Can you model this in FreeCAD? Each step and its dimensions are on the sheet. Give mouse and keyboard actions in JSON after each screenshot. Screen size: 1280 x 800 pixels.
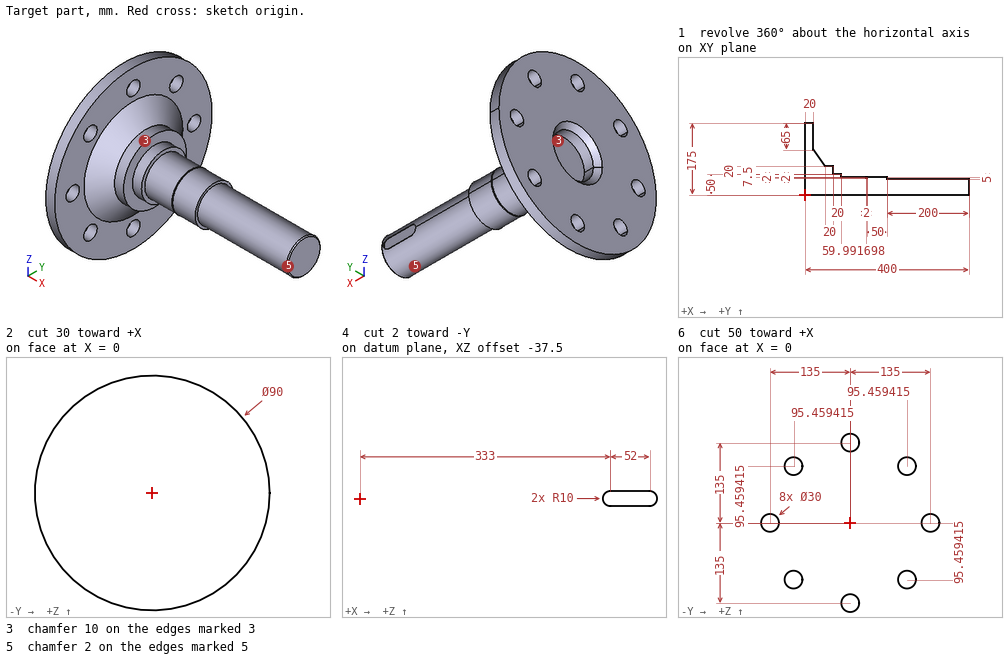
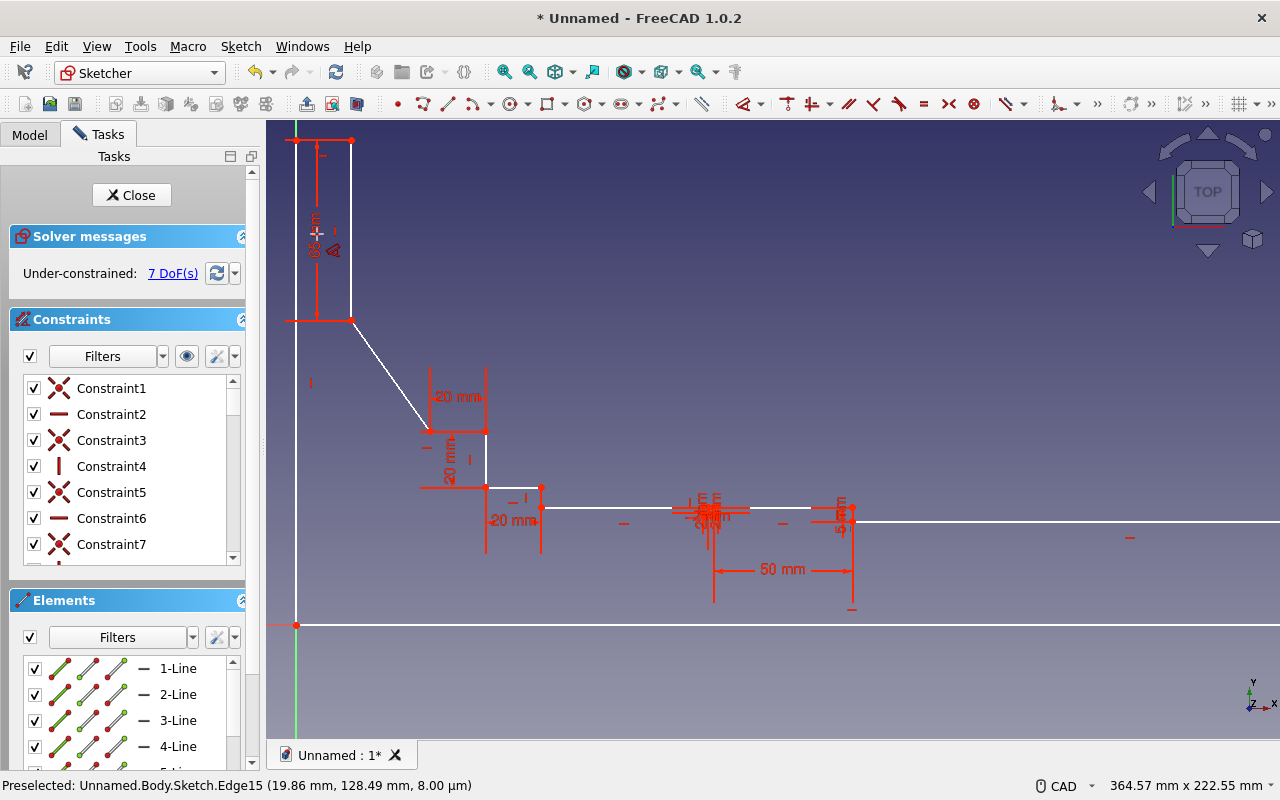
{"action": "scroll", "coordinate": [525, 487], "scroll_direction": "down", "scroll_amount": 3}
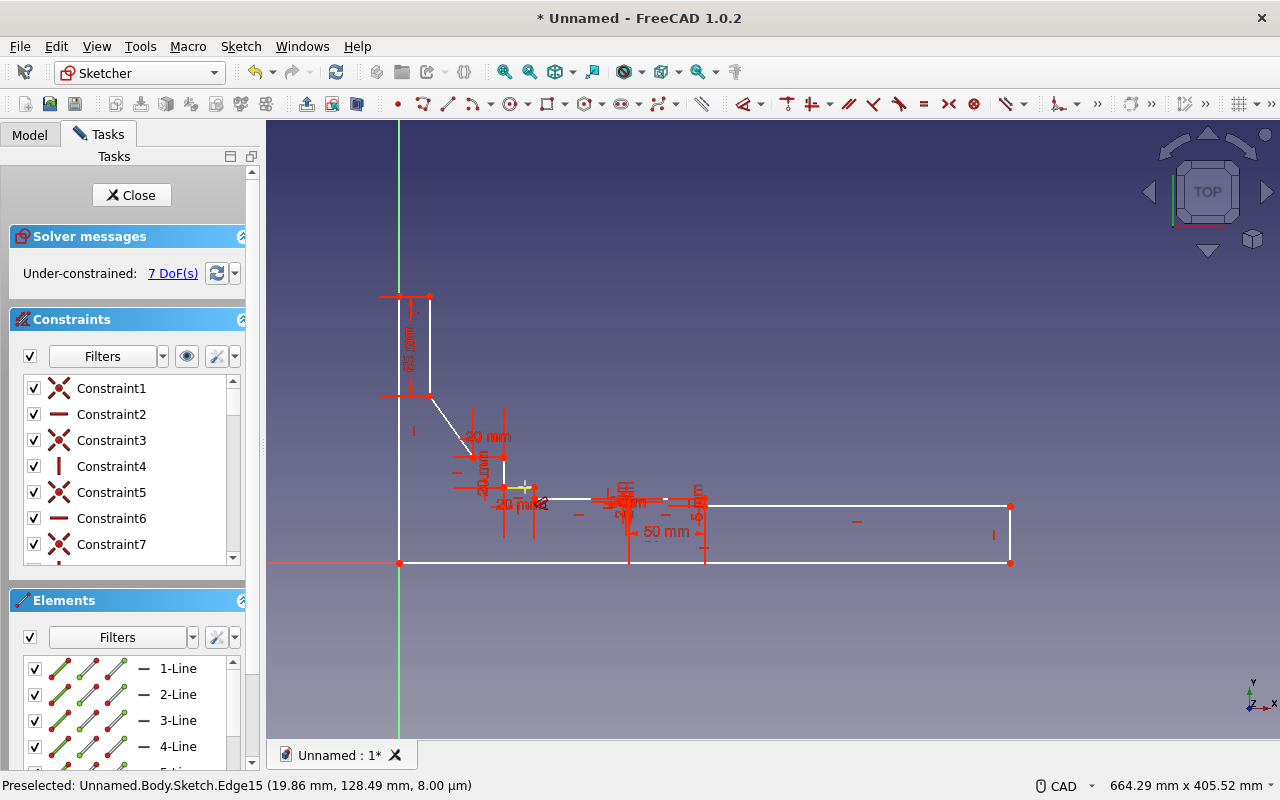
{"action": "scroll", "coordinate": [421, 297], "scroll_direction": "up", "scroll_amount": 3}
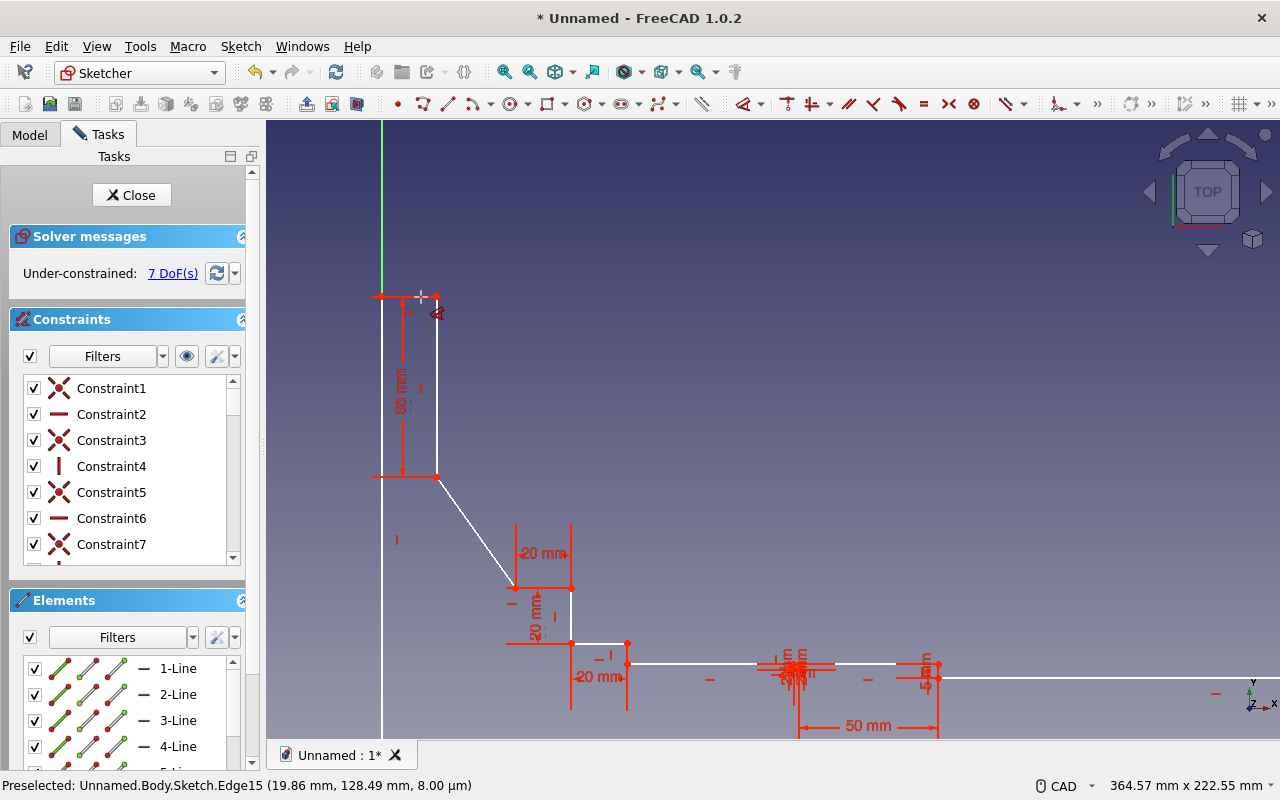
{"action": "left_click", "coordinate": [420, 297]}
{"action": "left_click", "coordinate": [409, 263]}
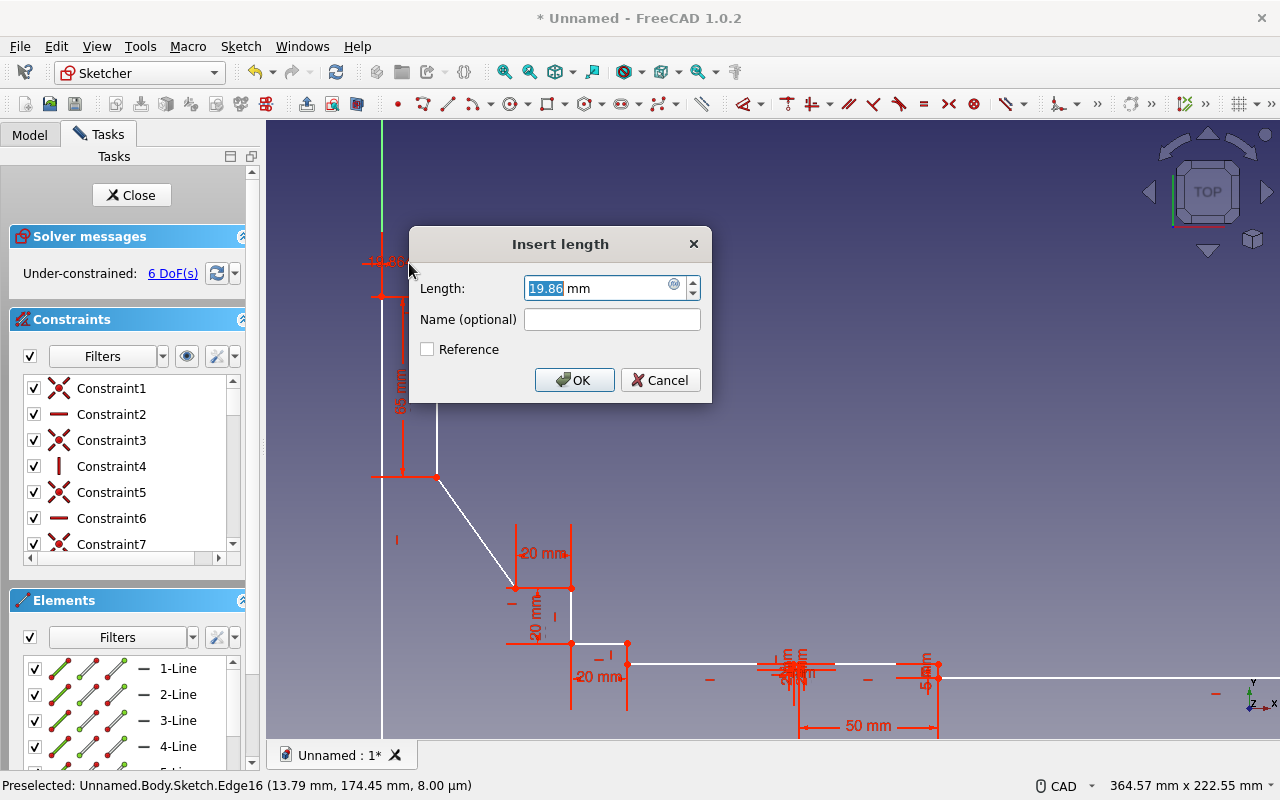
{"action": "type", "text": "20"}
{"action": "key", "text": "Return"}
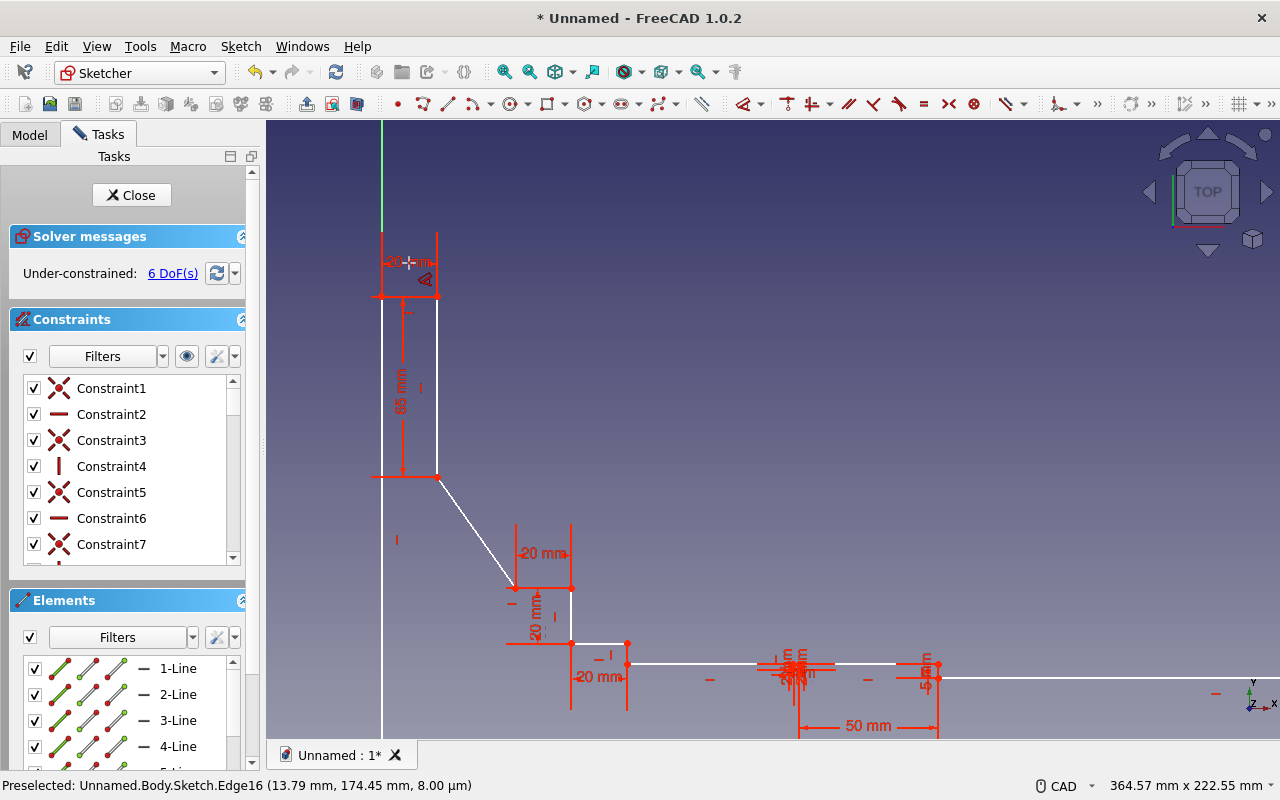
{"action": "scroll", "coordinate": [421, 297], "scroll_direction": "down", "scroll_amount": 3}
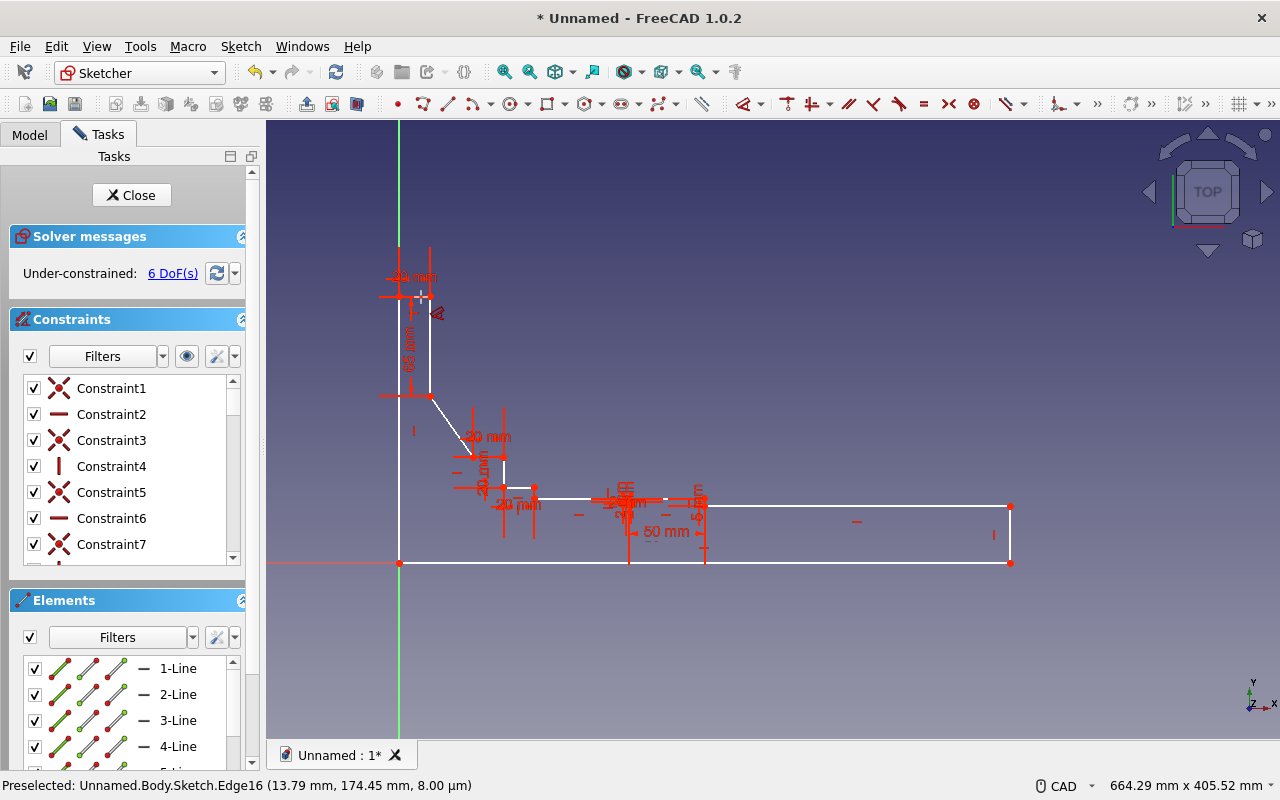
{"action": "left_click", "coordinate": [583, 563]}
{"action": "left_click", "coordinate": [705, 597]}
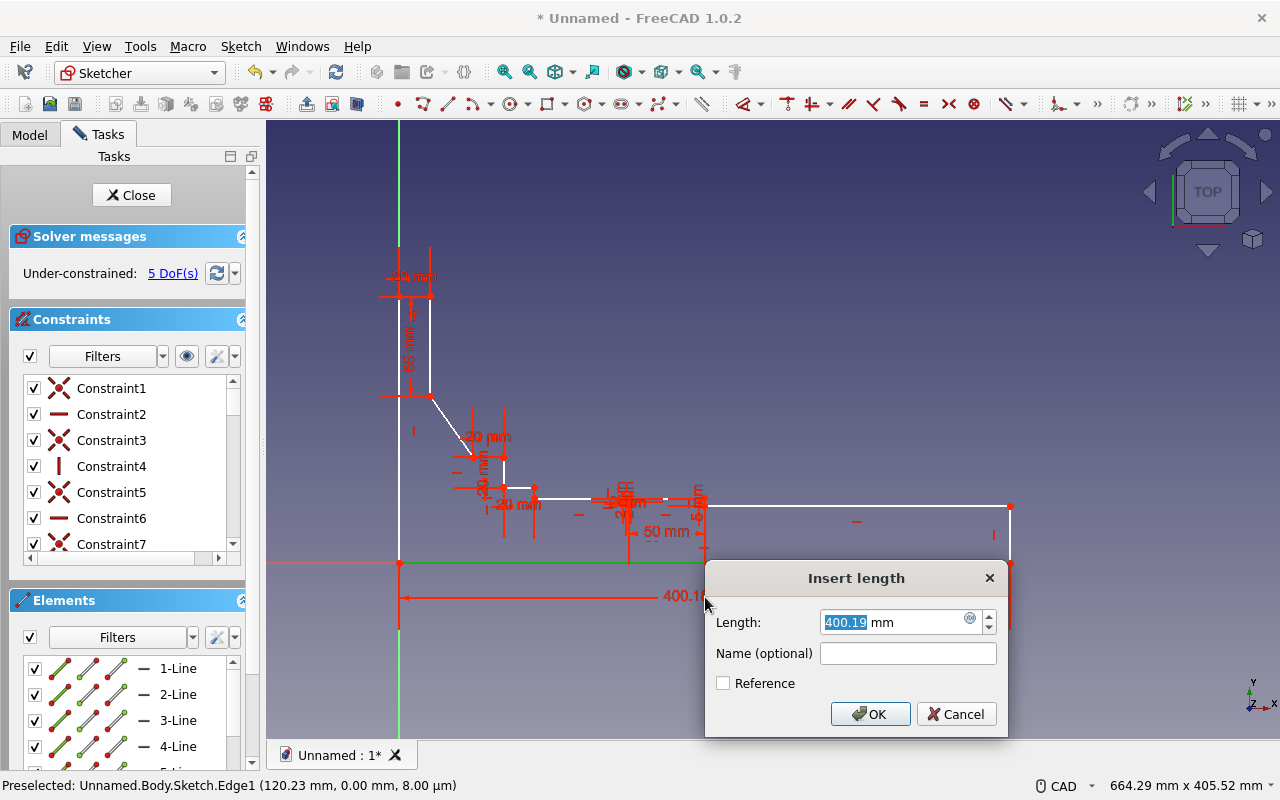
{"action": "type", "text": "400"}
{"action": "key", "text": "Return"}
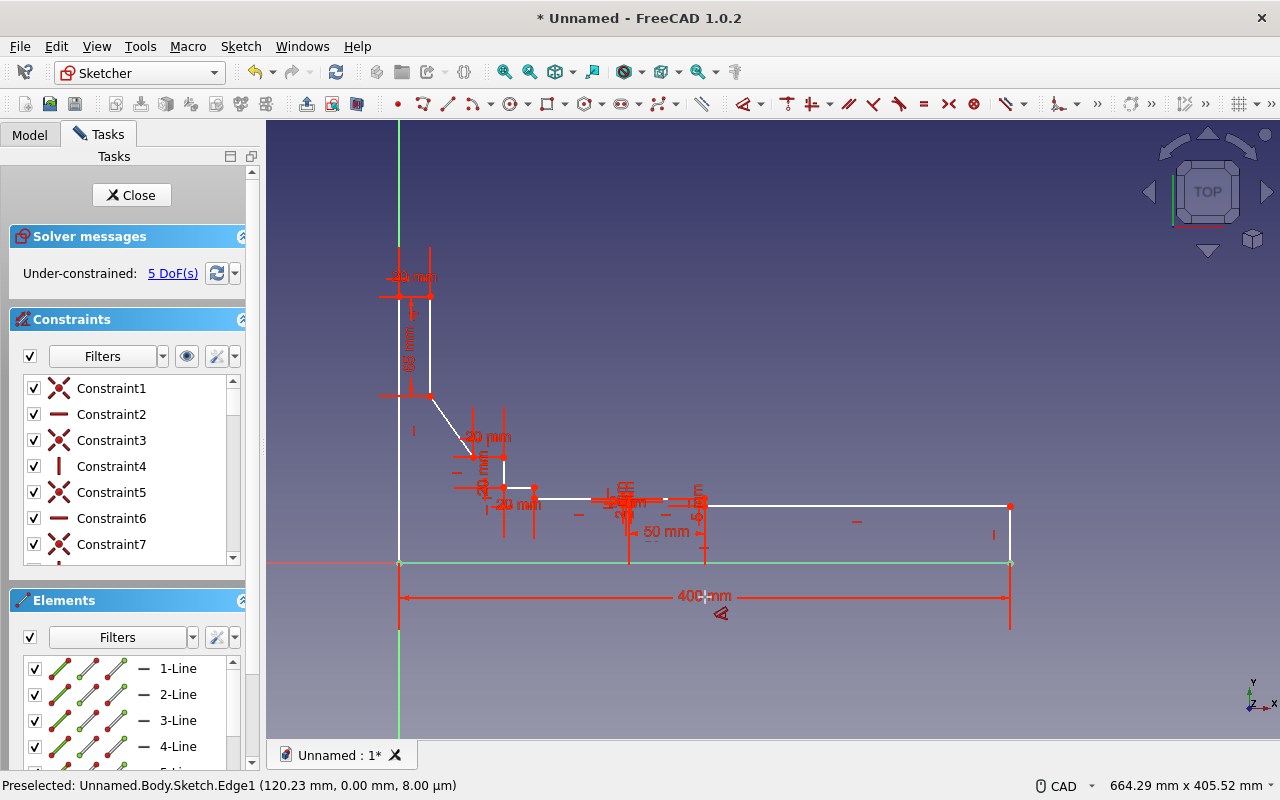
{"action": "left_click", "coordinate": [919, 506]}
{"action": "left_click", "coordinate": [857, 540]}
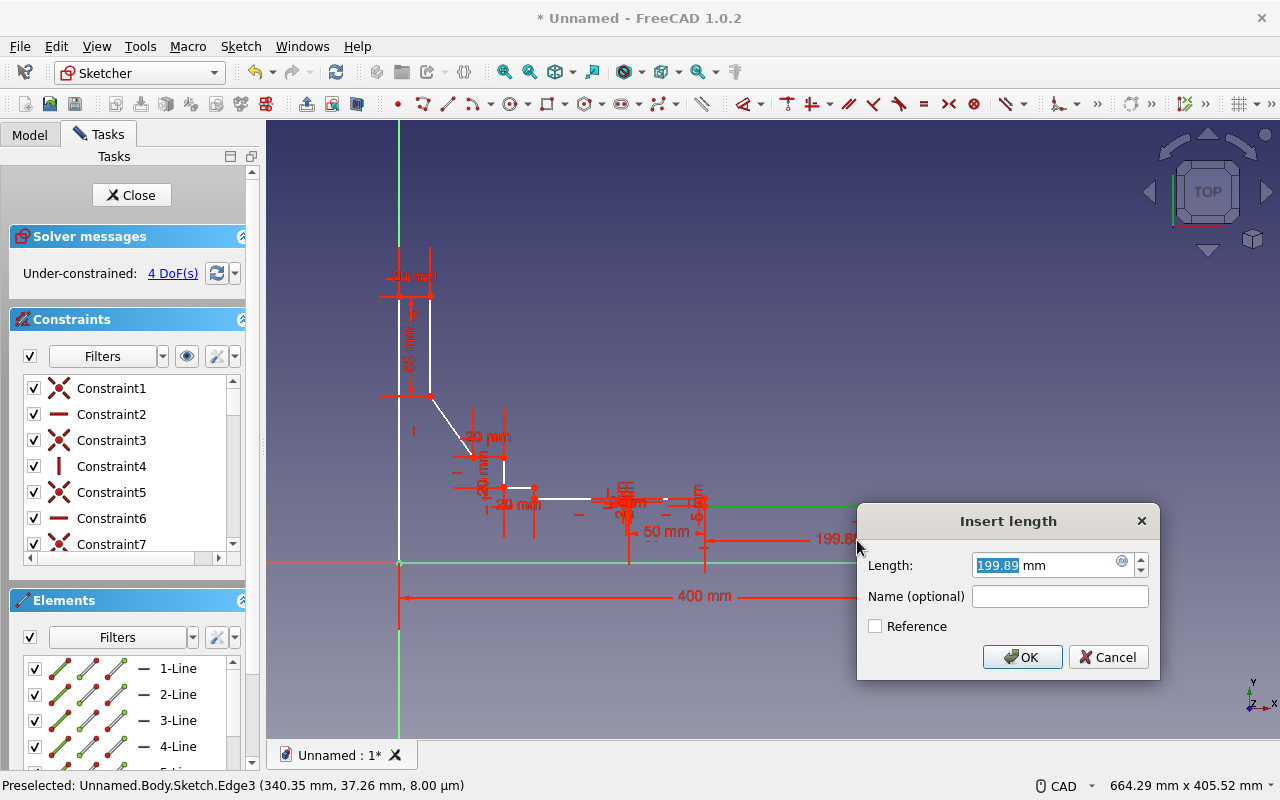
{"action": "type", "text": "200"}
{"action": "key", "text": "Return"}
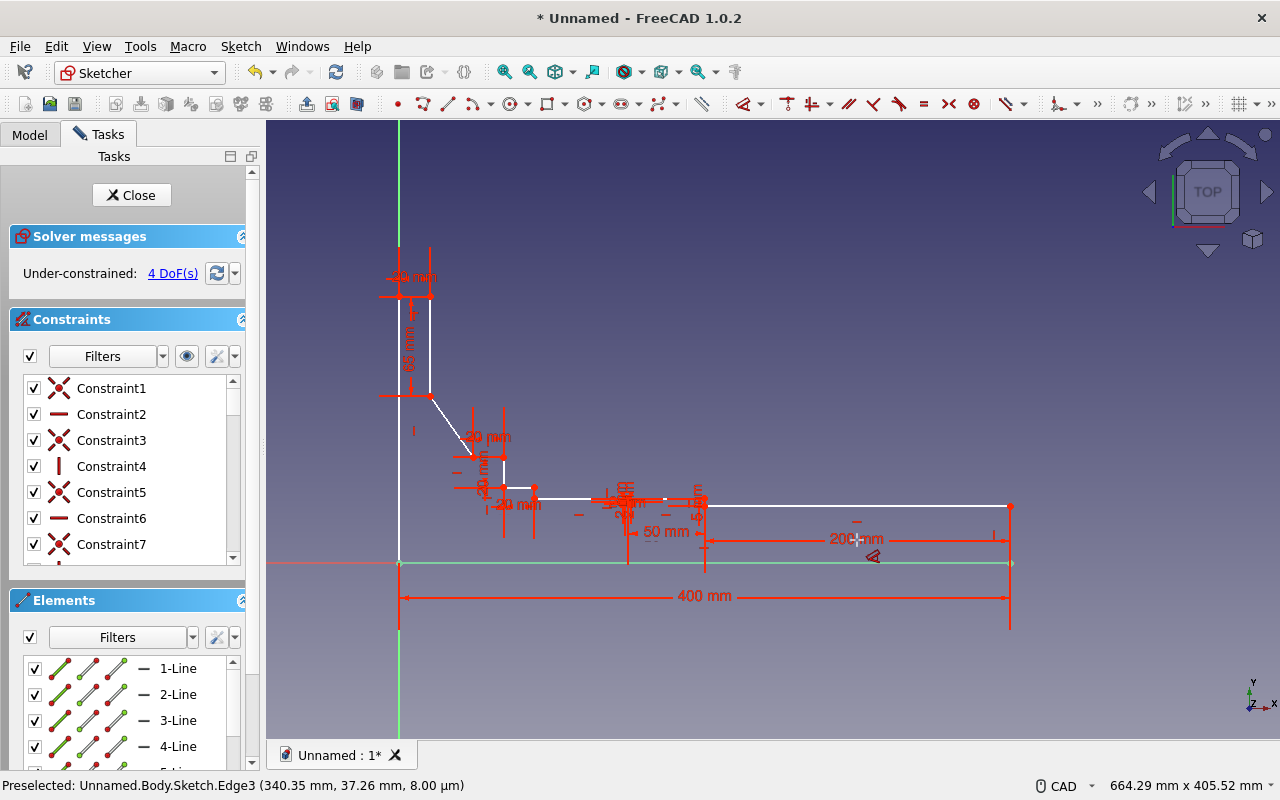
{"action": "scroll", "coordinate": [534, 493], "scroll_direction": "up", "scroll_amount": 7}